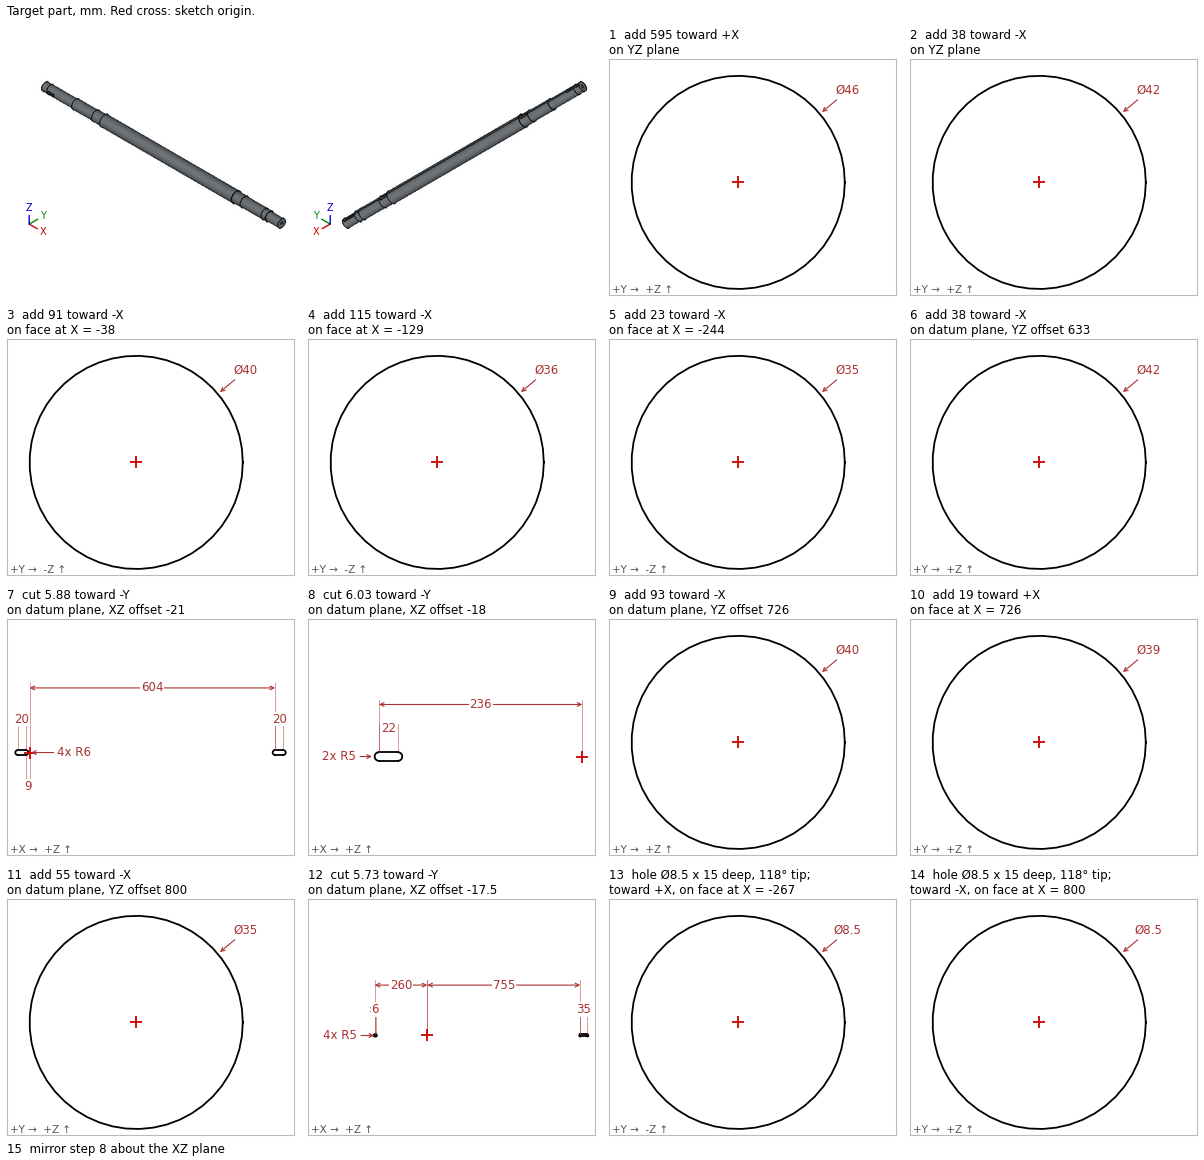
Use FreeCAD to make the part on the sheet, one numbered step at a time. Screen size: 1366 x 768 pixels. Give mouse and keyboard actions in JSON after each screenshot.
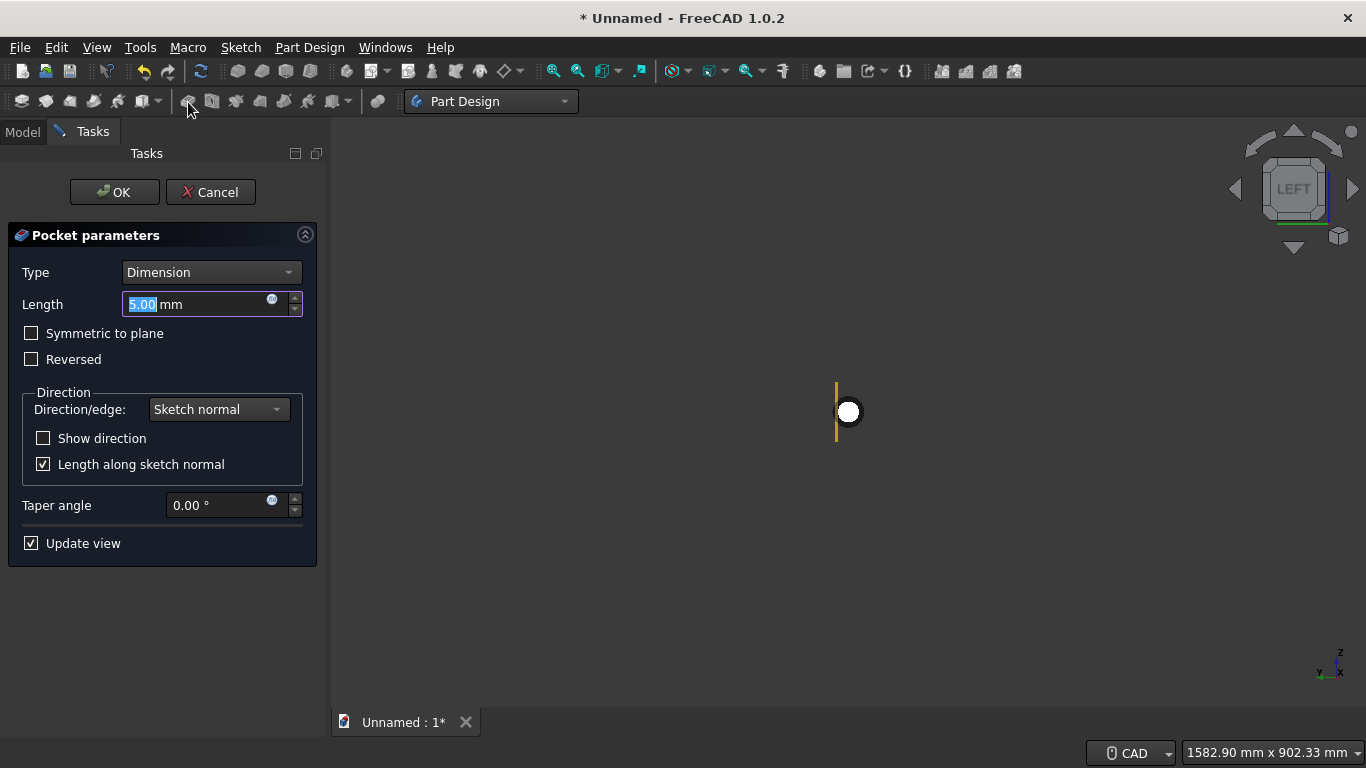
{"action": "type", "text": "6.03"}
{"action": "key", "text": "Tab"}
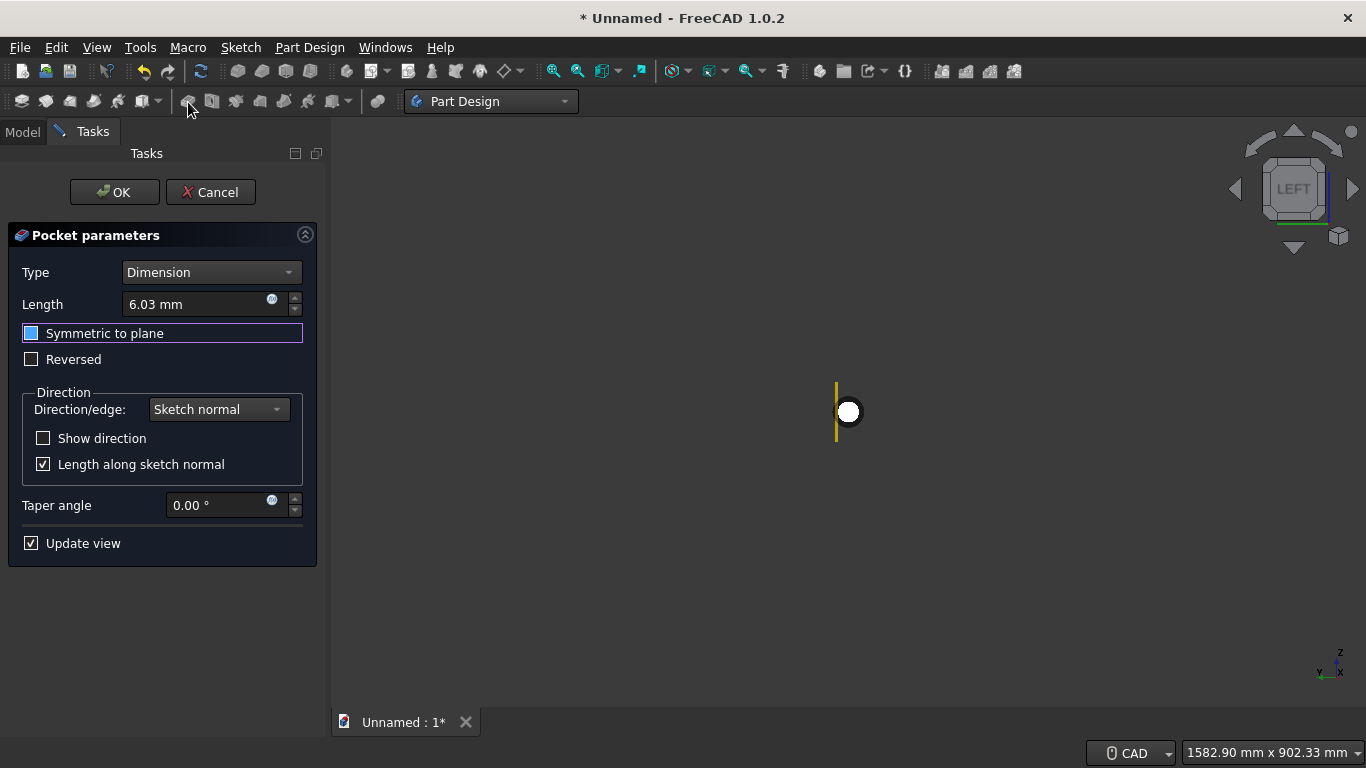
{"action": "left_click", "coordinate": [30, 359]}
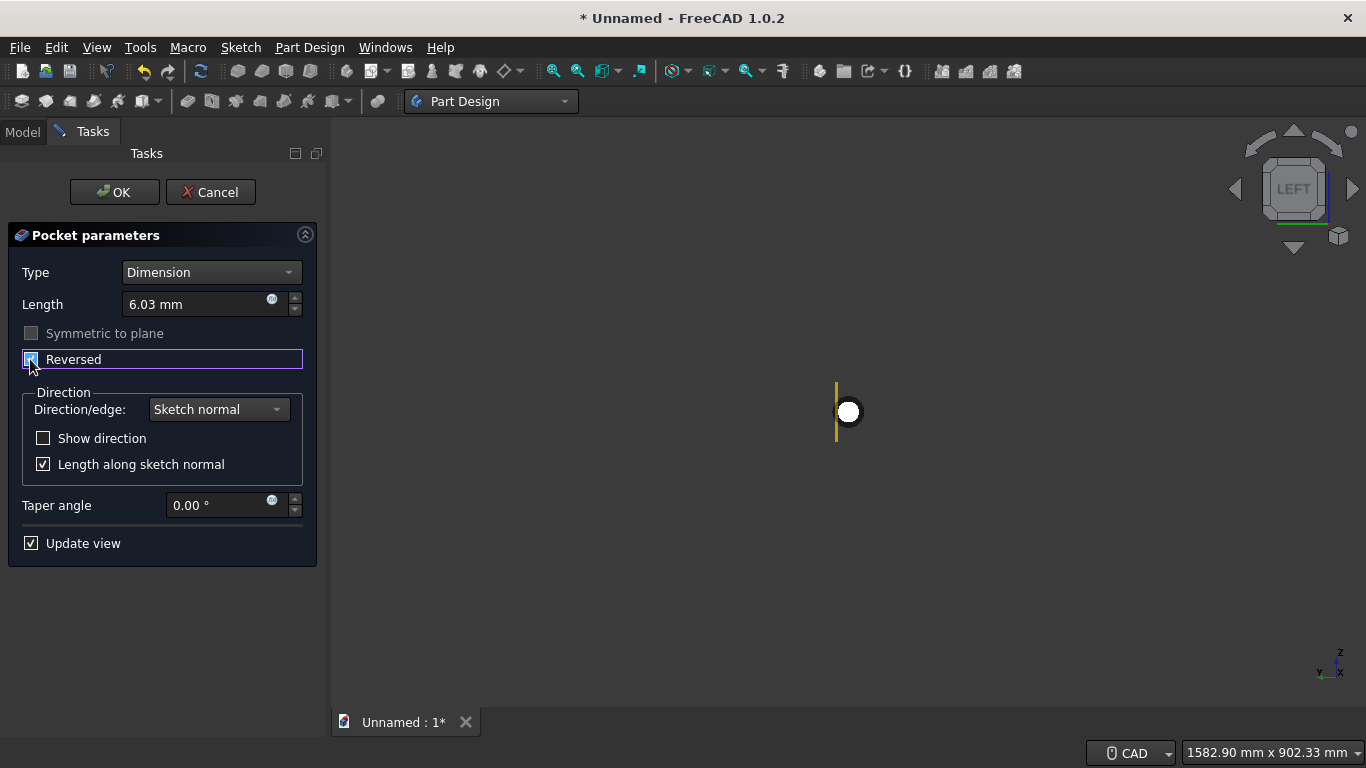
{"action": "left_click", "coordinate": [115, 192]}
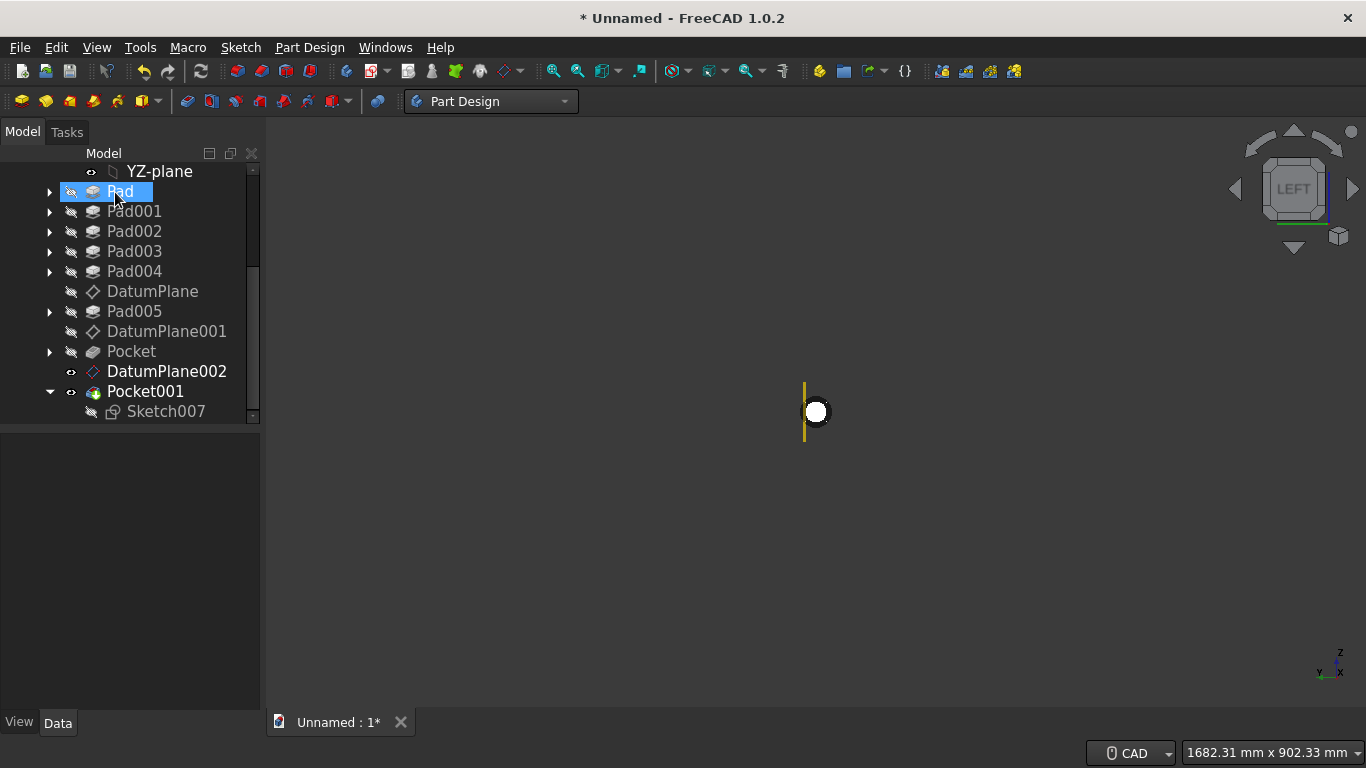
{"action": "left_click", "coordinate": [116, 372]}
{"action": "key", "text": "space"}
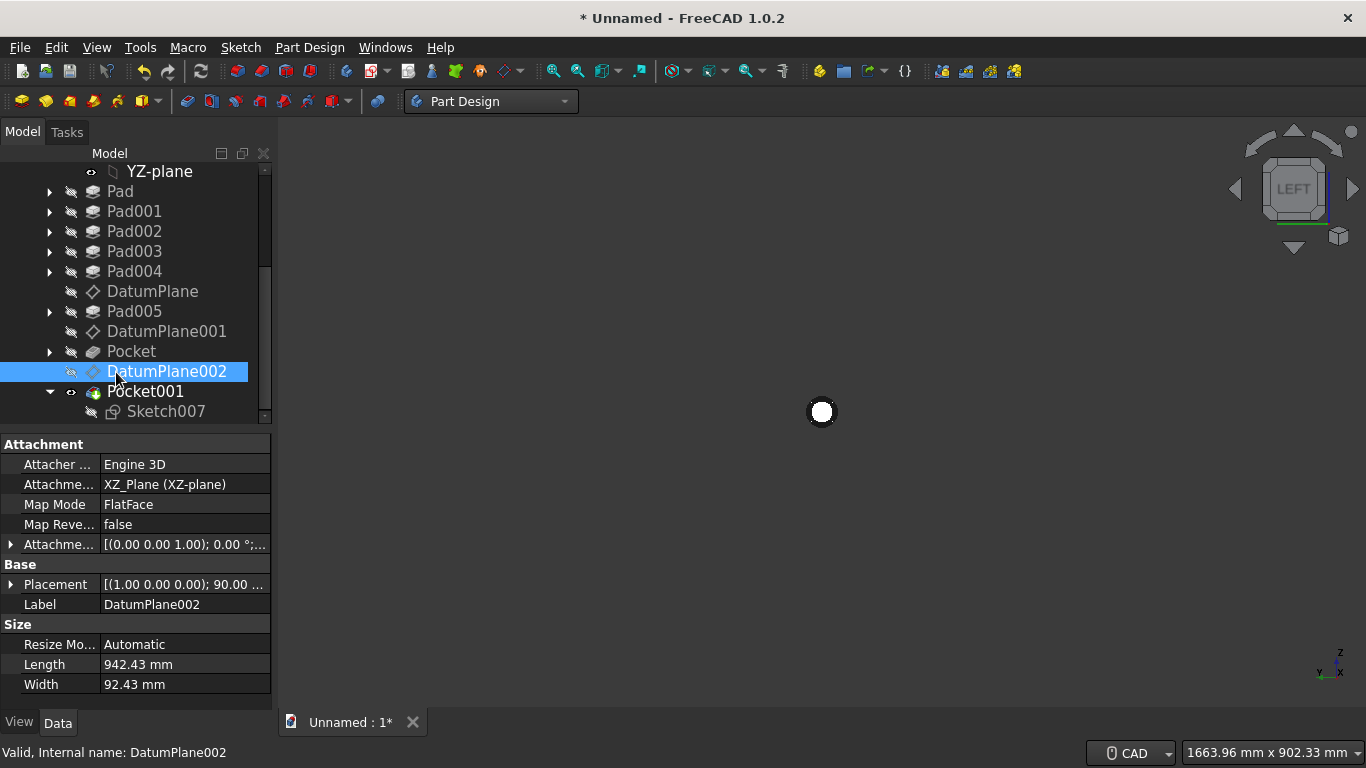
{"action": "key", "text": "v f"}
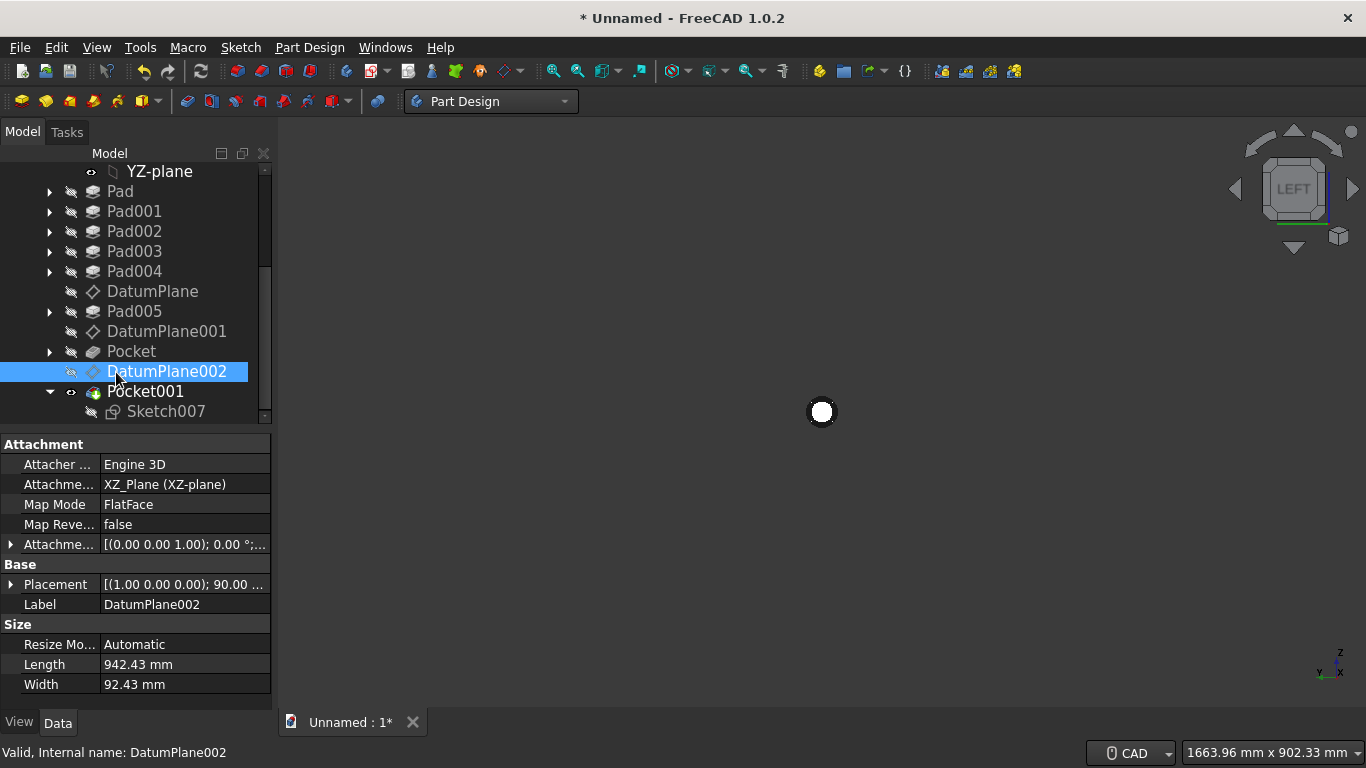
{"action": "scroll", "coordinate": [160, 287], "scroll_direction": "down", "scroll_amount": 3}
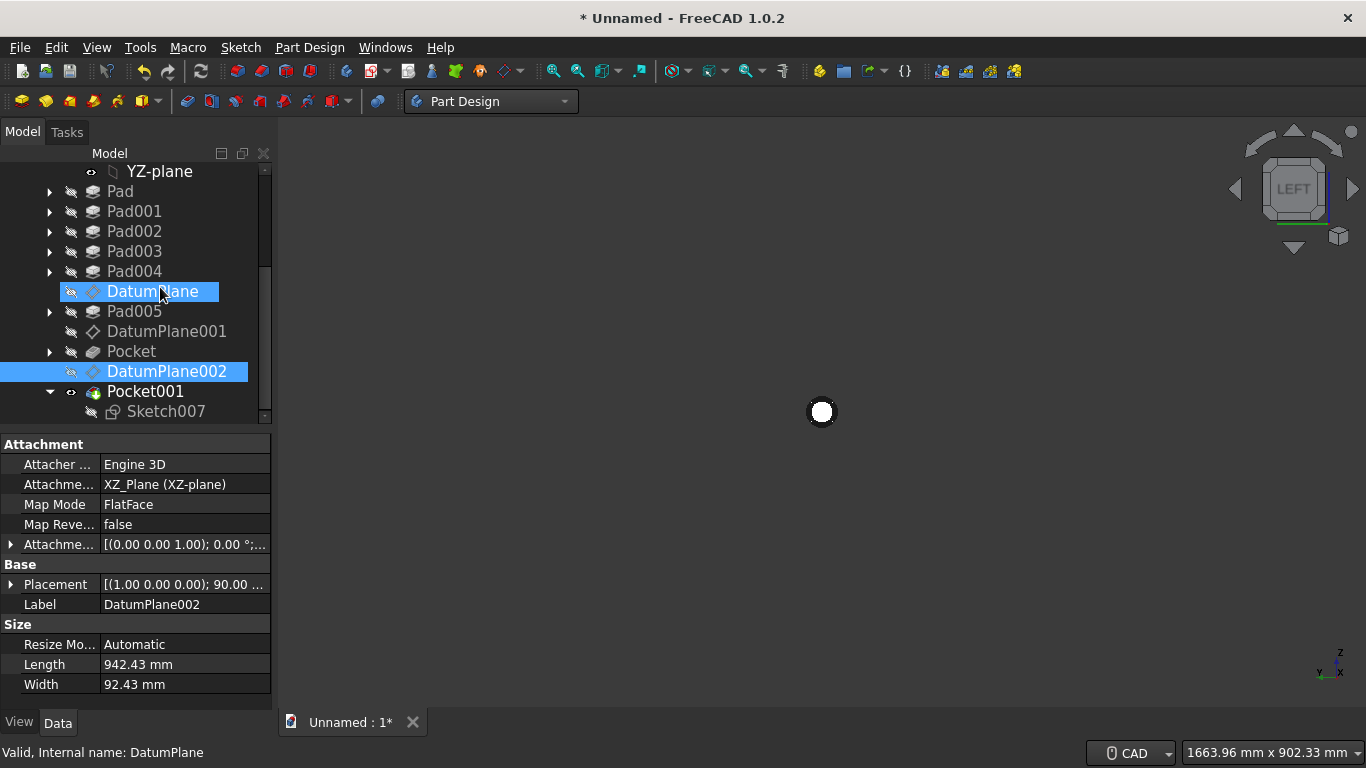
{"action": "scroll", "coordinate": [160, 287], "scroll_direction": "up", "scroll_amount": 15}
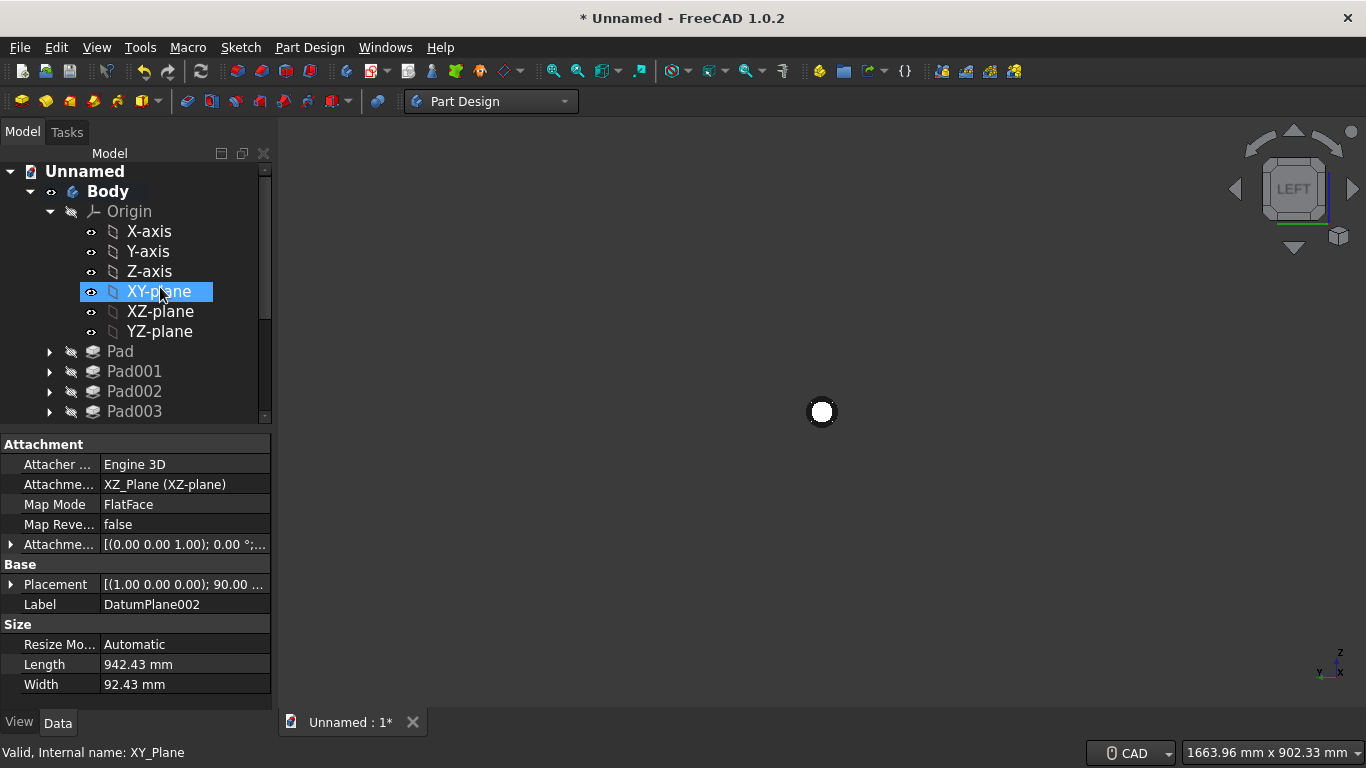
{"action": "left_click", "coordinate": [136, 332]}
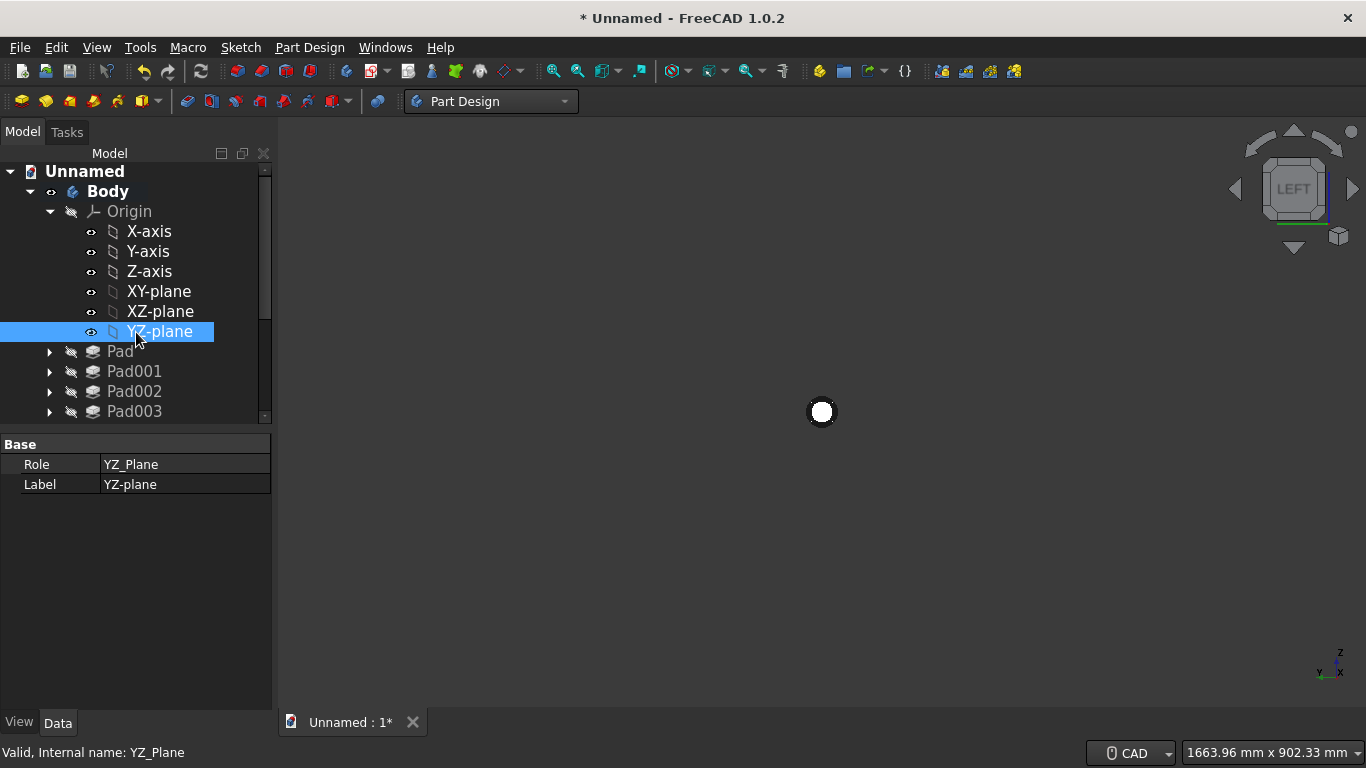
{"action": "left_click", "coordinate": [504, 72]}